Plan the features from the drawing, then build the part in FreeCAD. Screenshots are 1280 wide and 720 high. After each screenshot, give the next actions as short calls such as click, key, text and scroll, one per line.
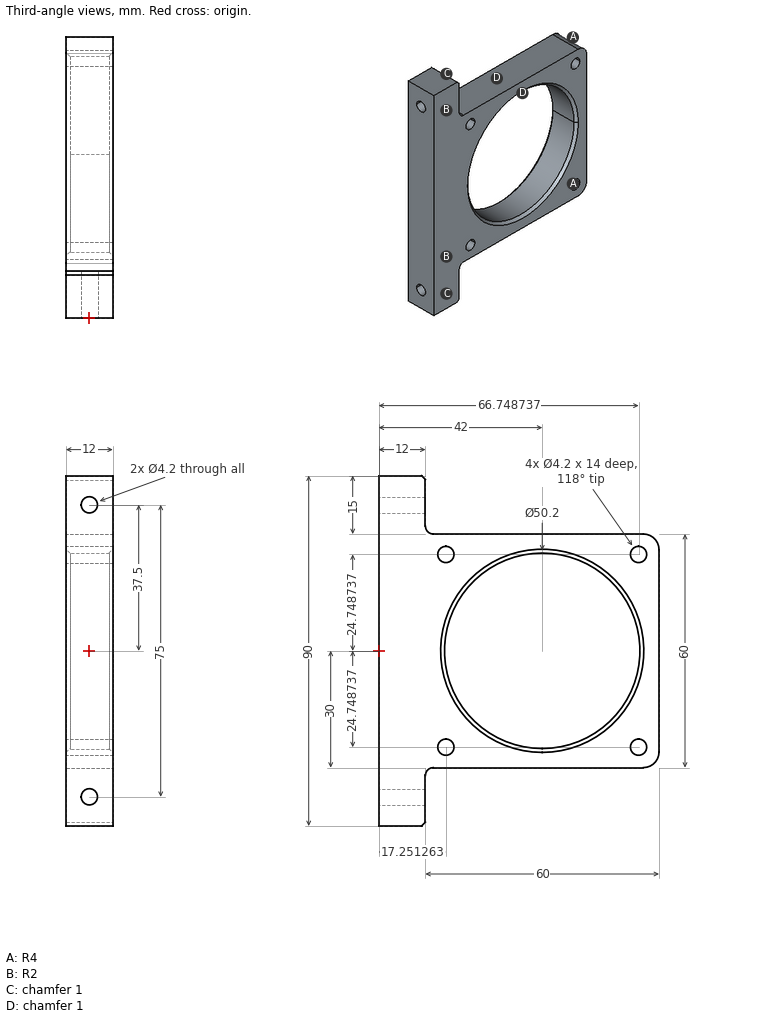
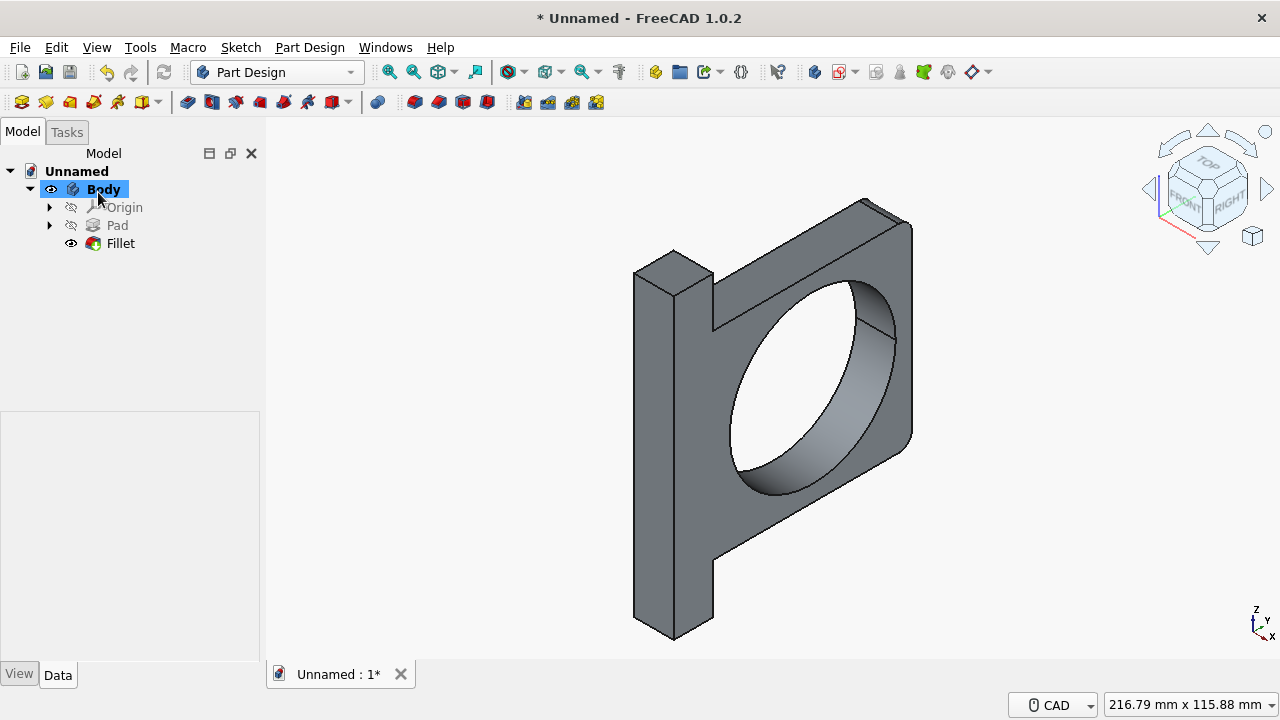
key(2)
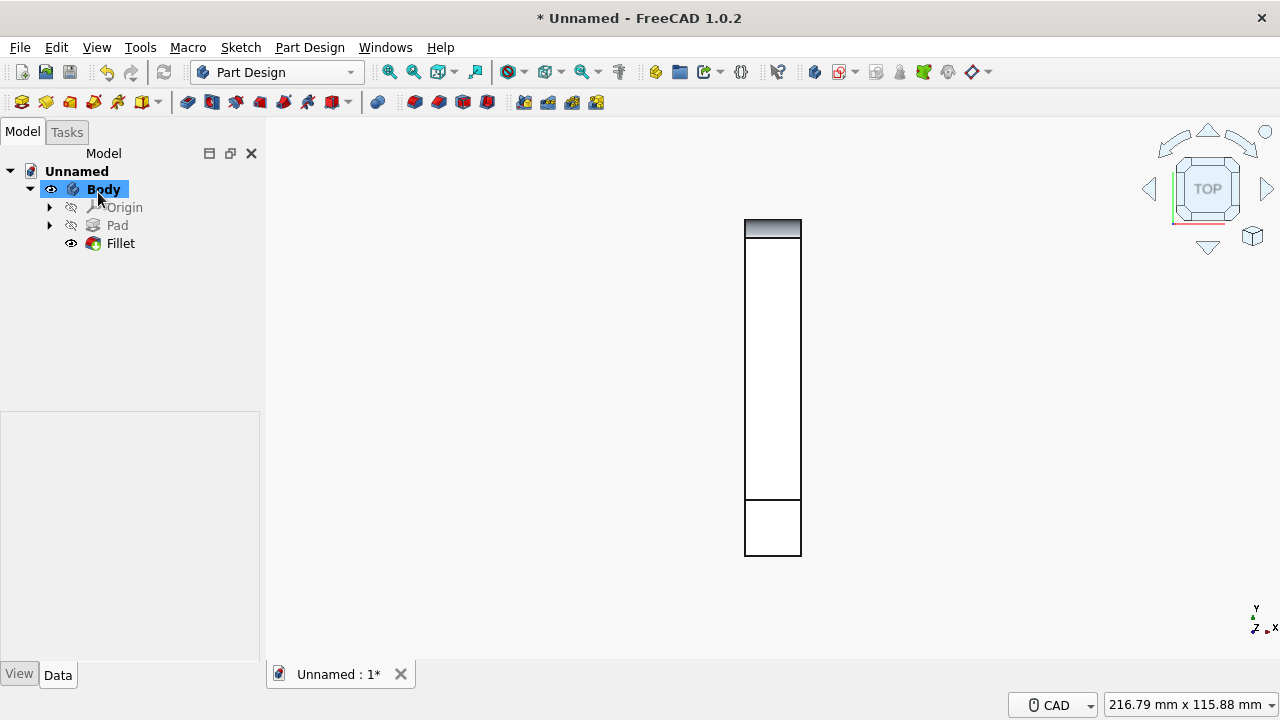
key(1)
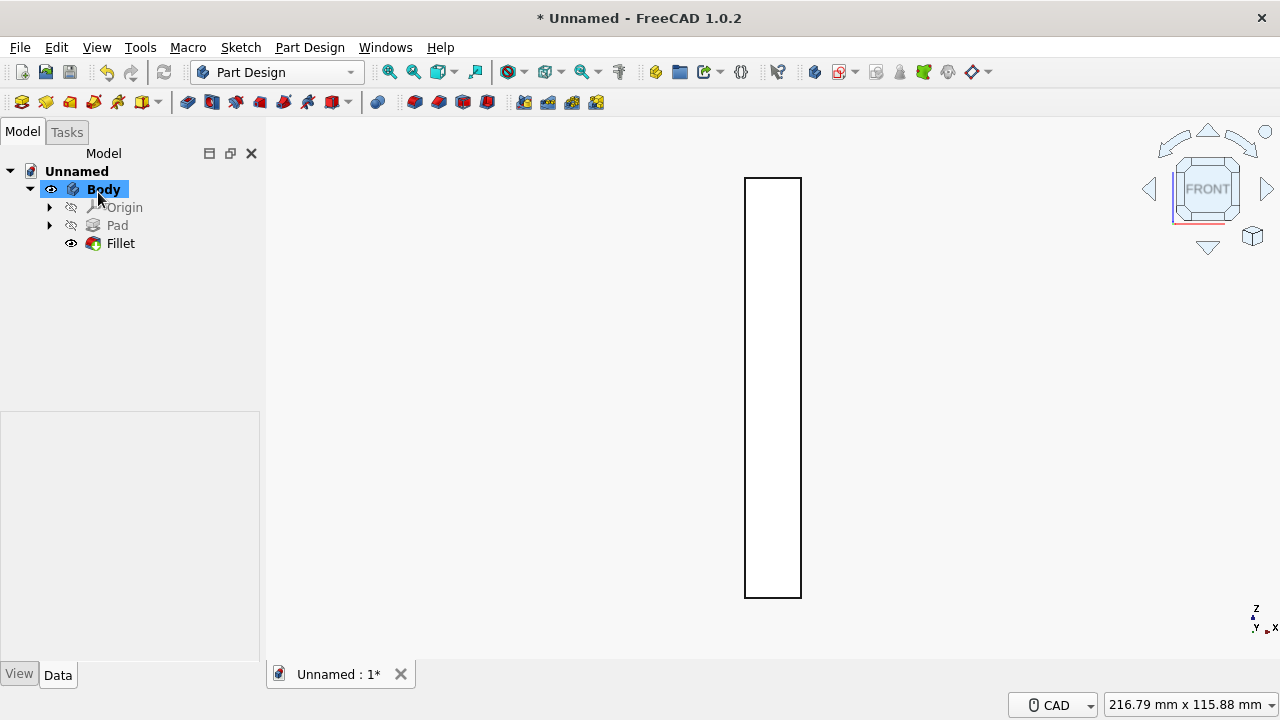
key(3)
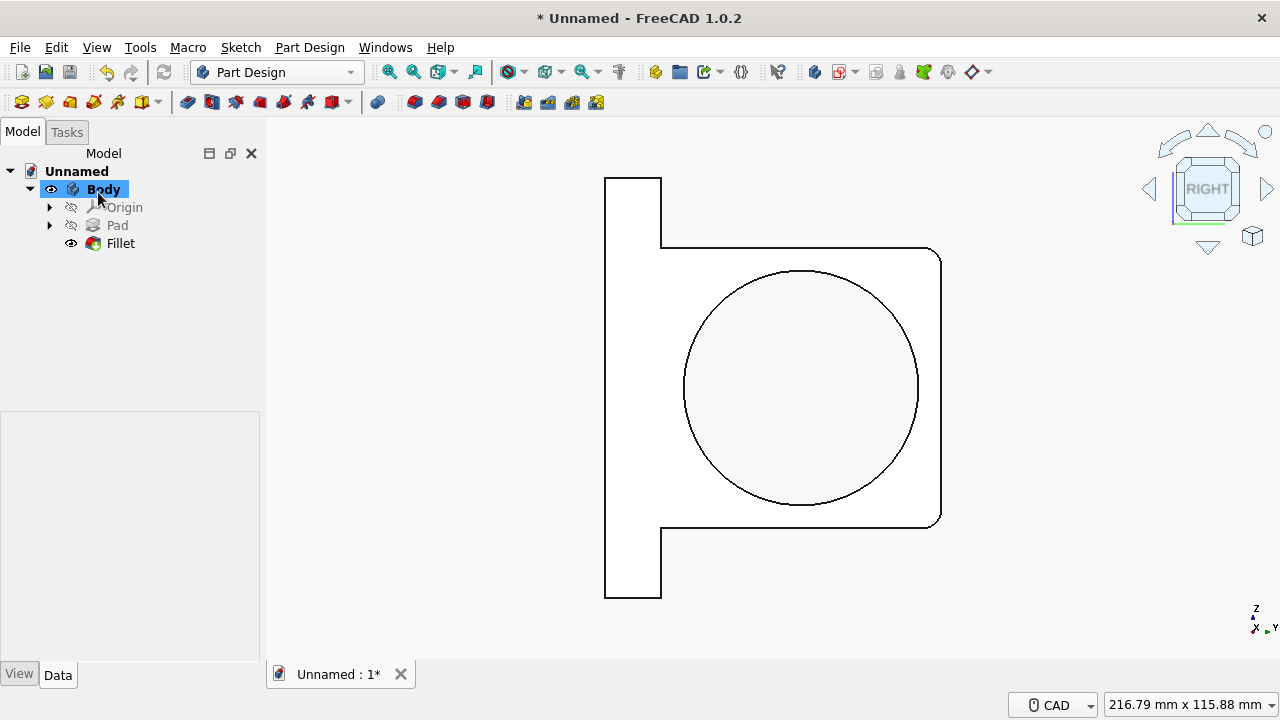
key(5)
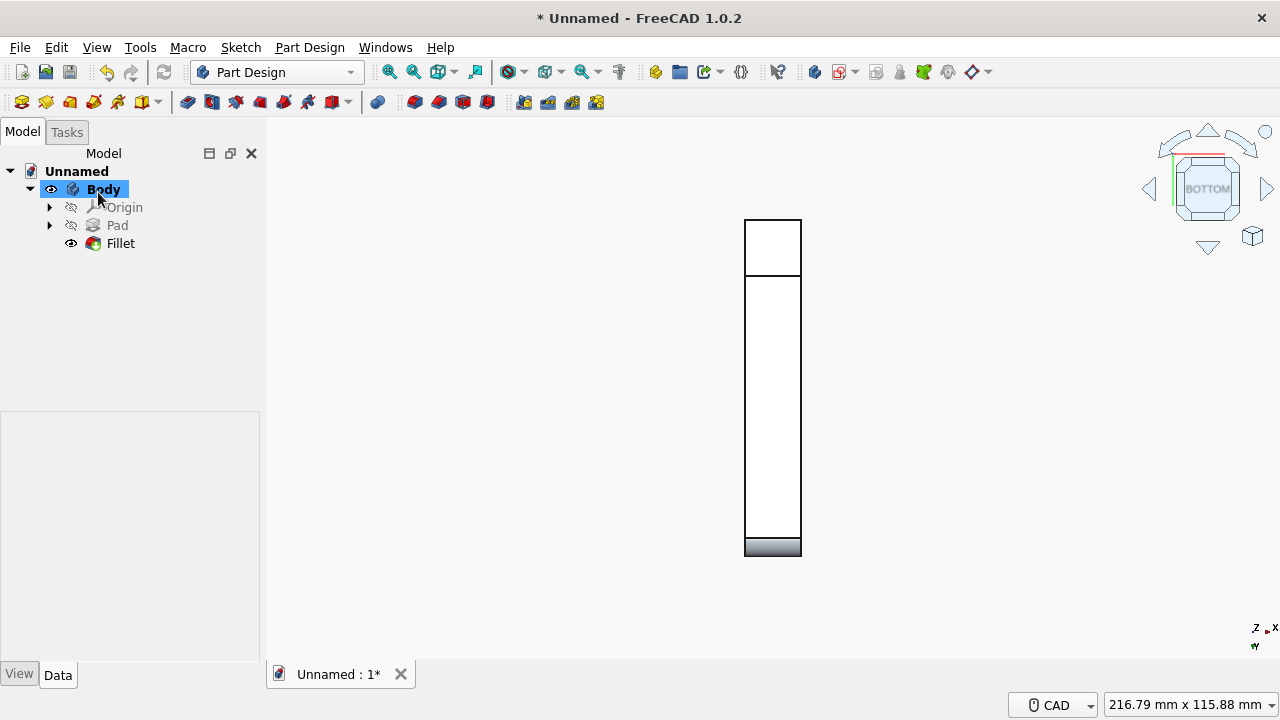
key(4)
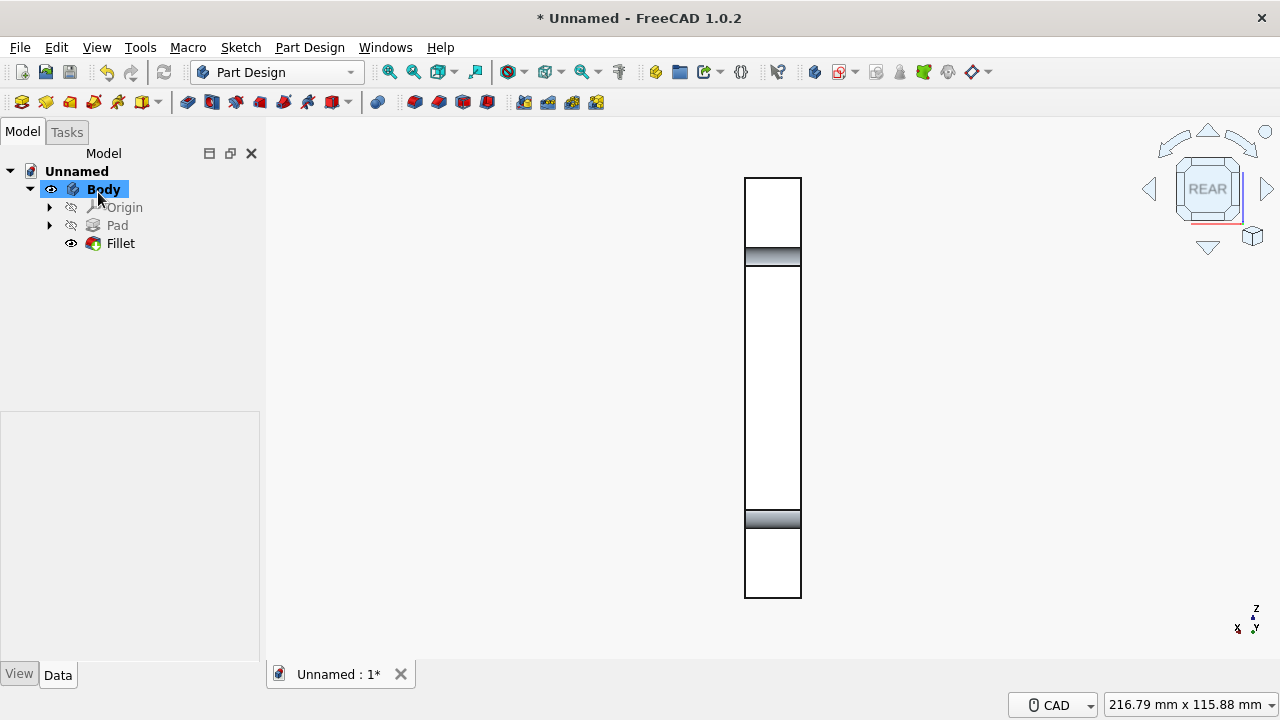
key(6)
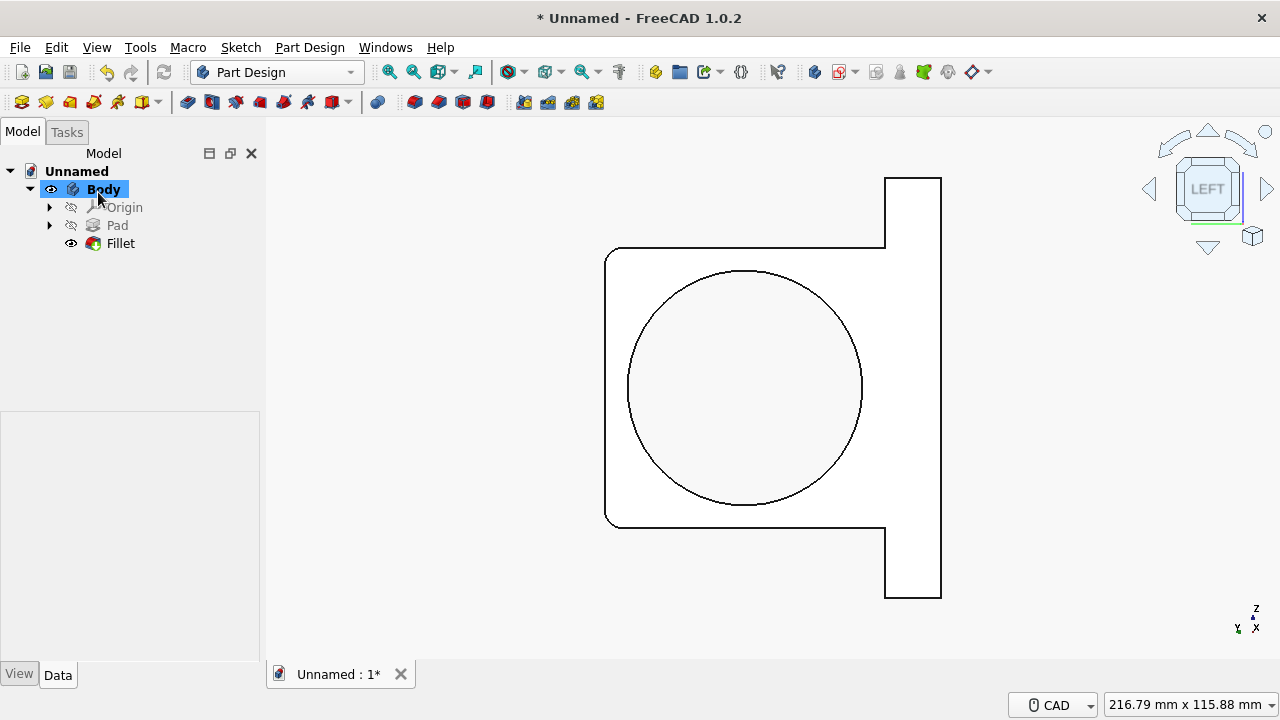
key(v)
key(3)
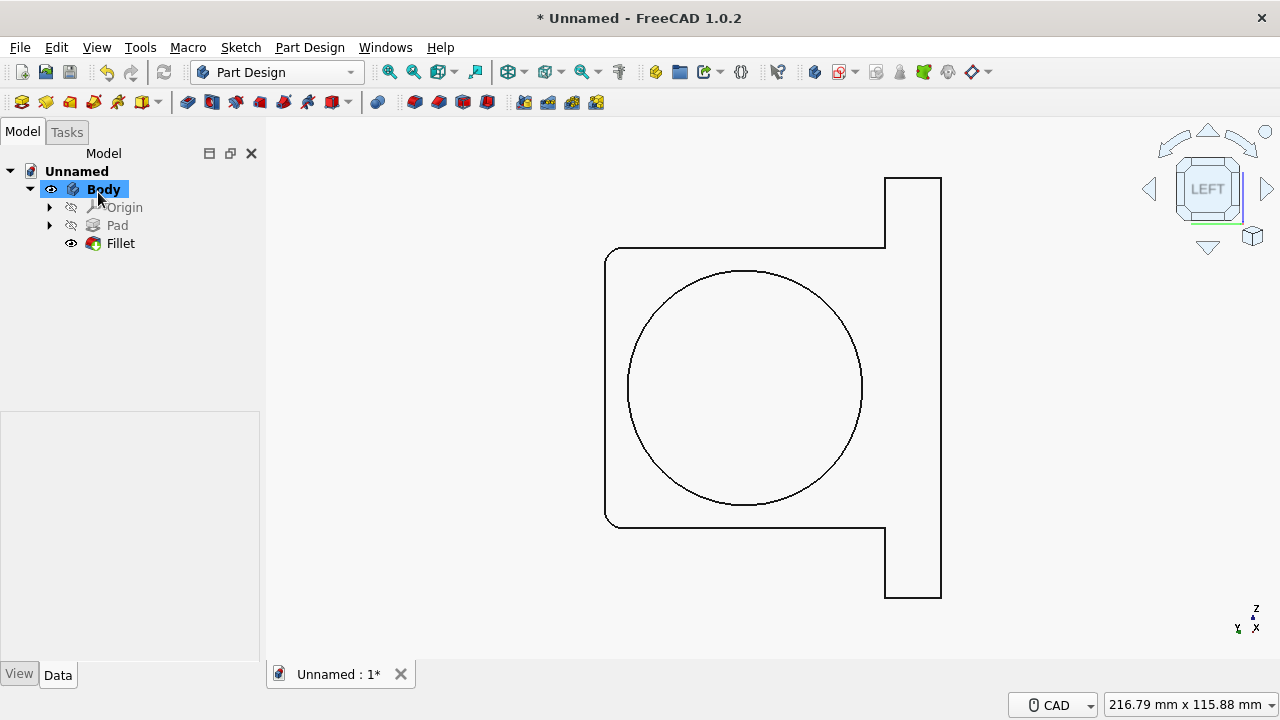
key(0)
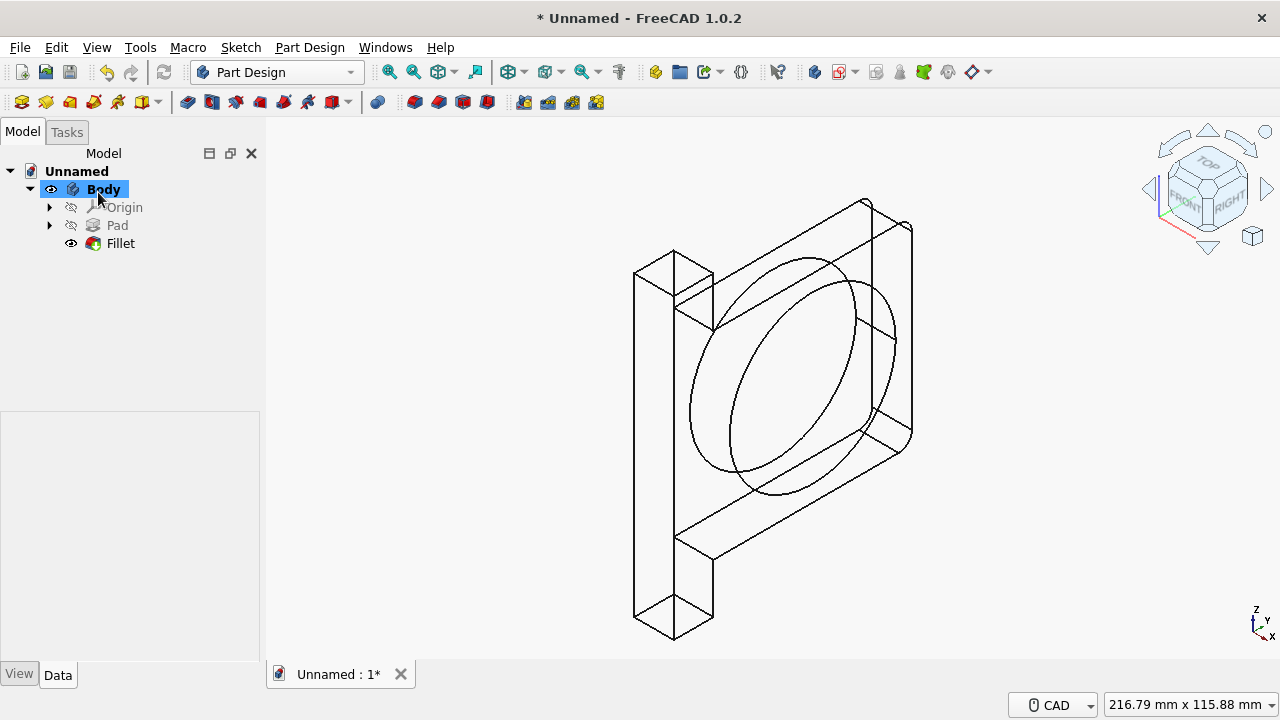
click(694, 318)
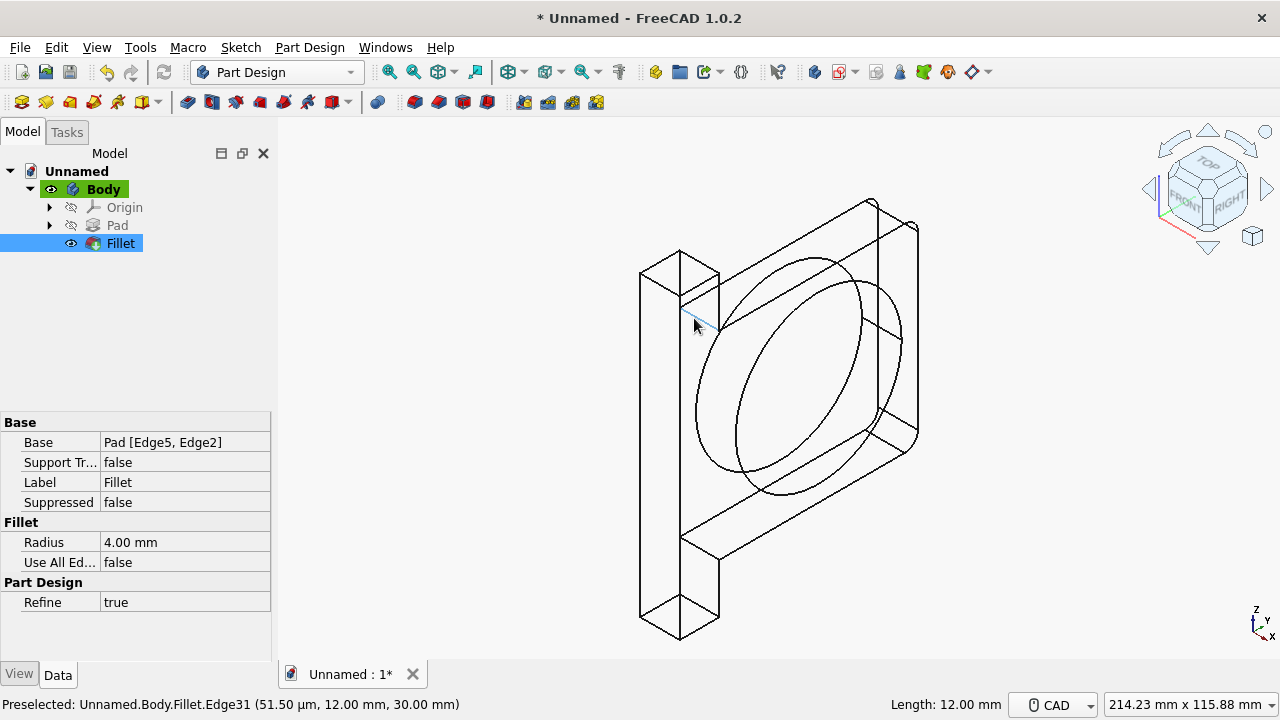
click(700, 547, ctrl)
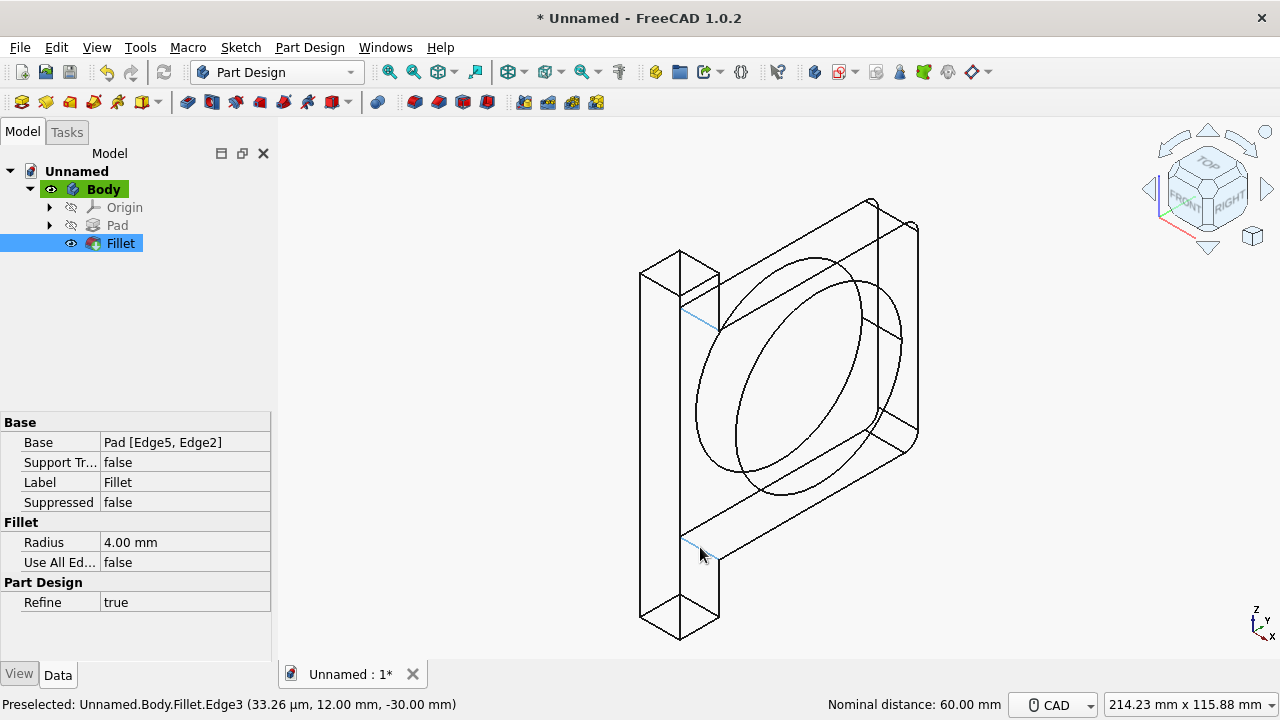
key(v)
key(1)